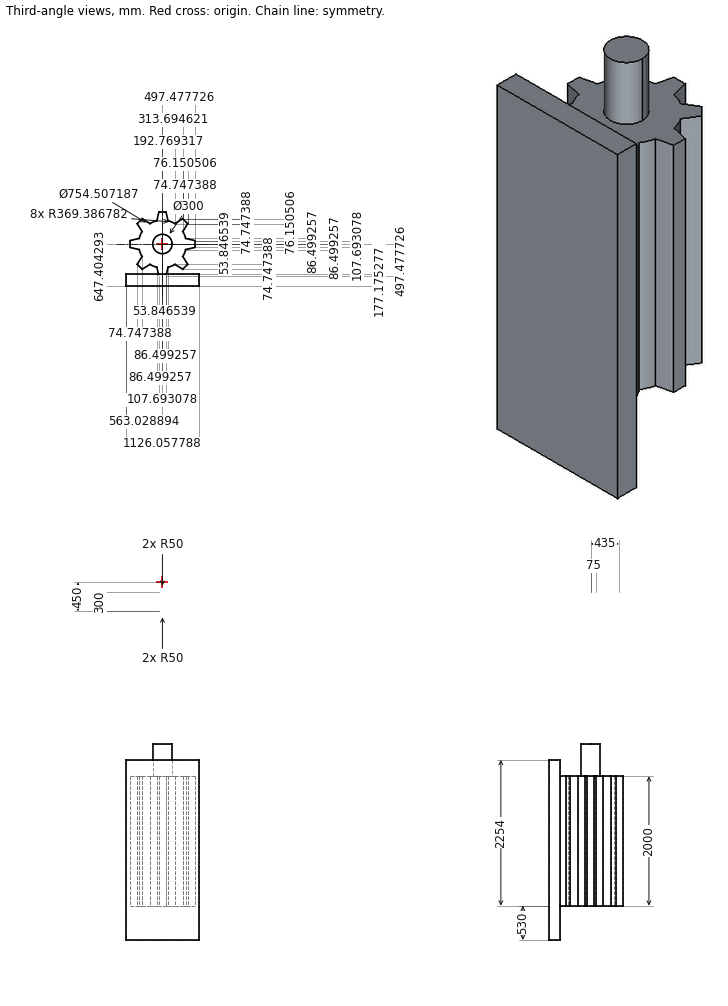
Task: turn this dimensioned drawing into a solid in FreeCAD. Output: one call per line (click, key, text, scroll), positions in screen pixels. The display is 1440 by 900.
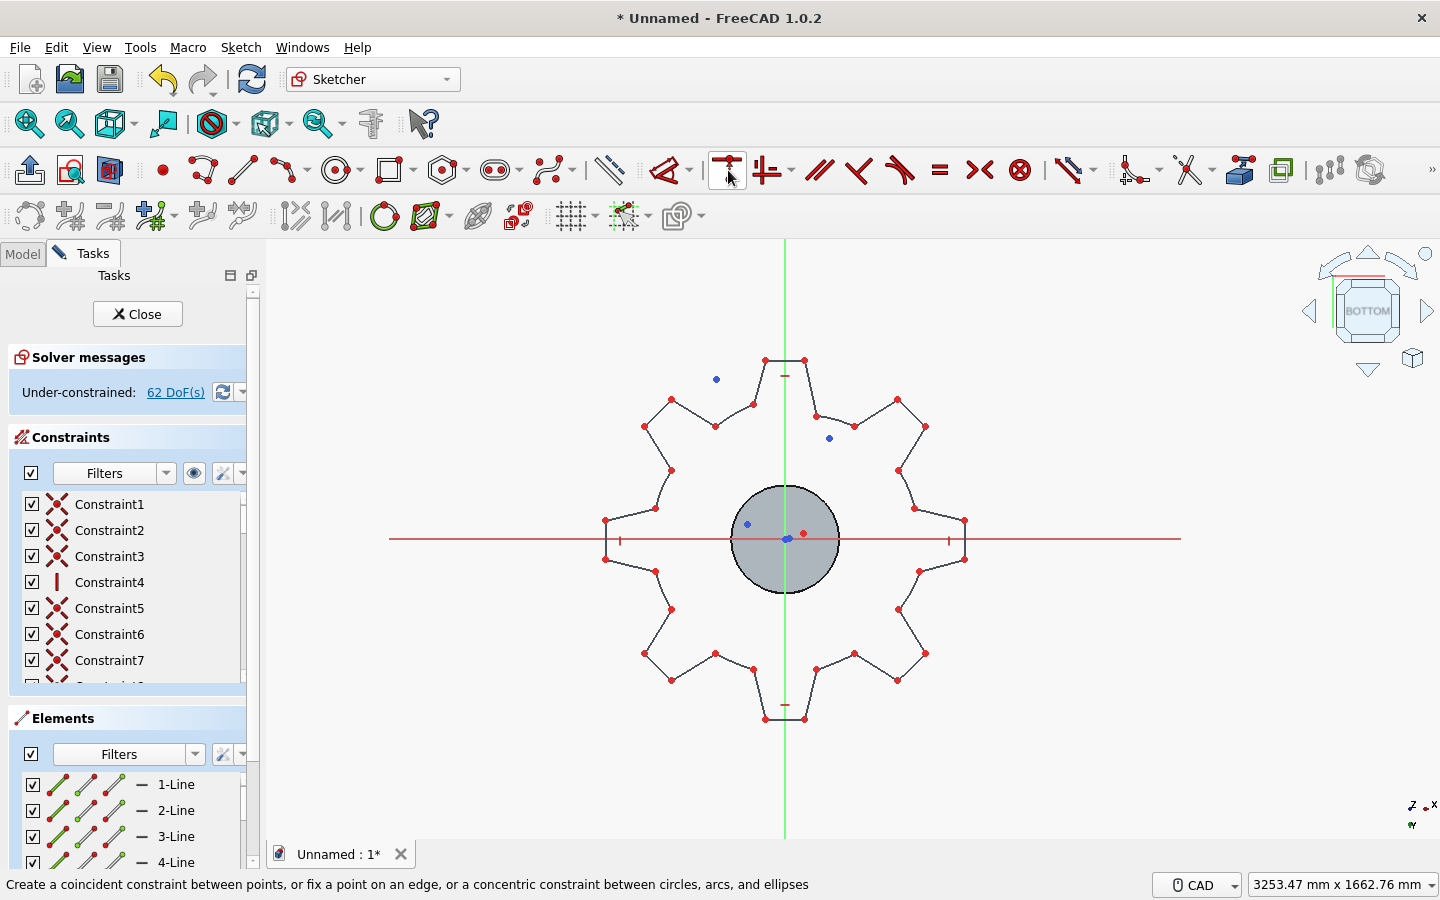
click(907, 599)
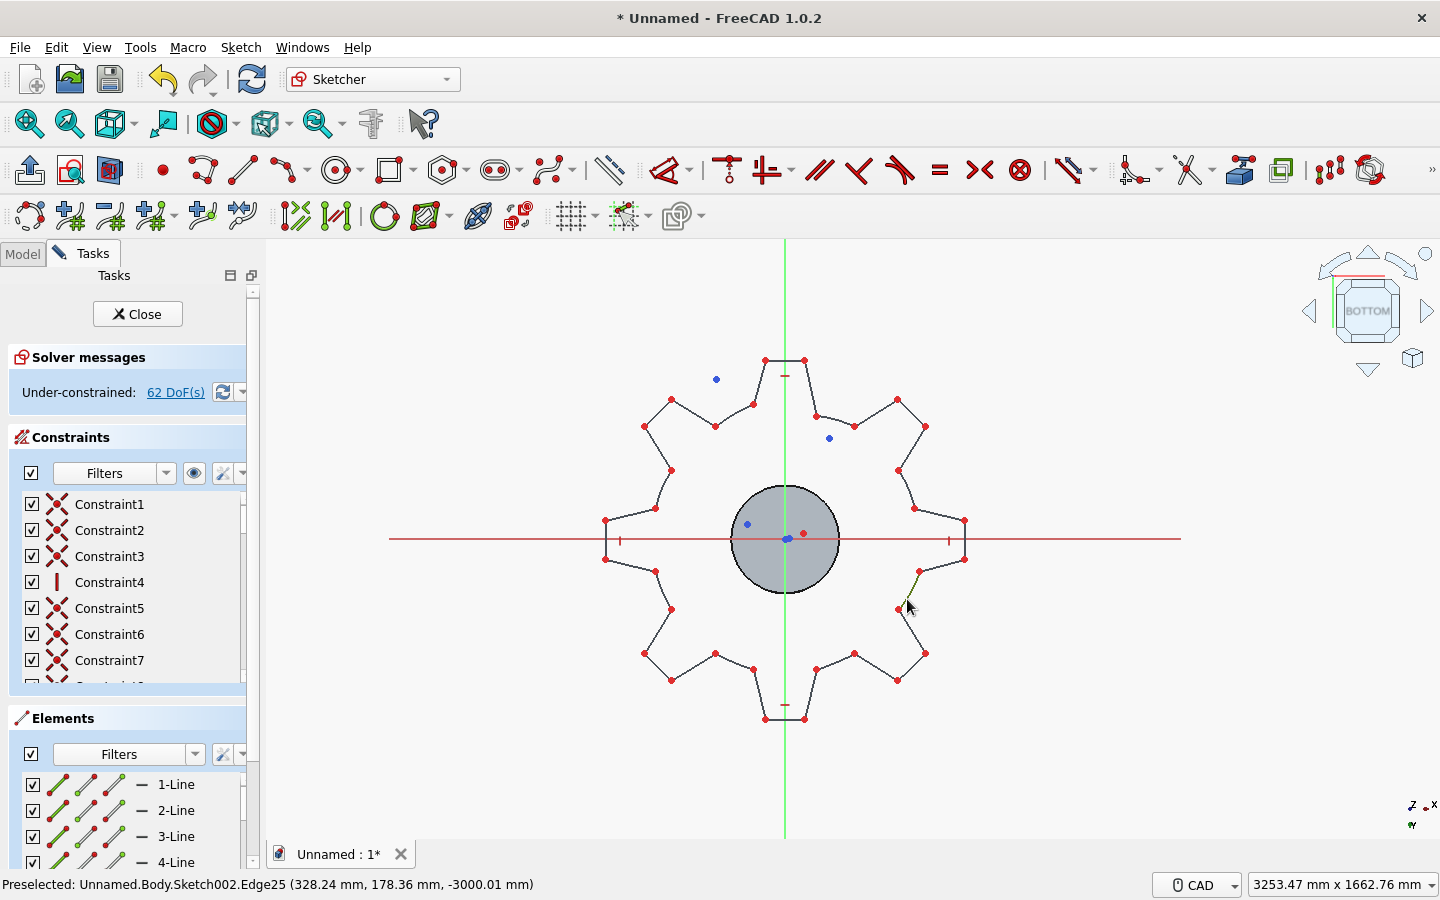
click(665, 481)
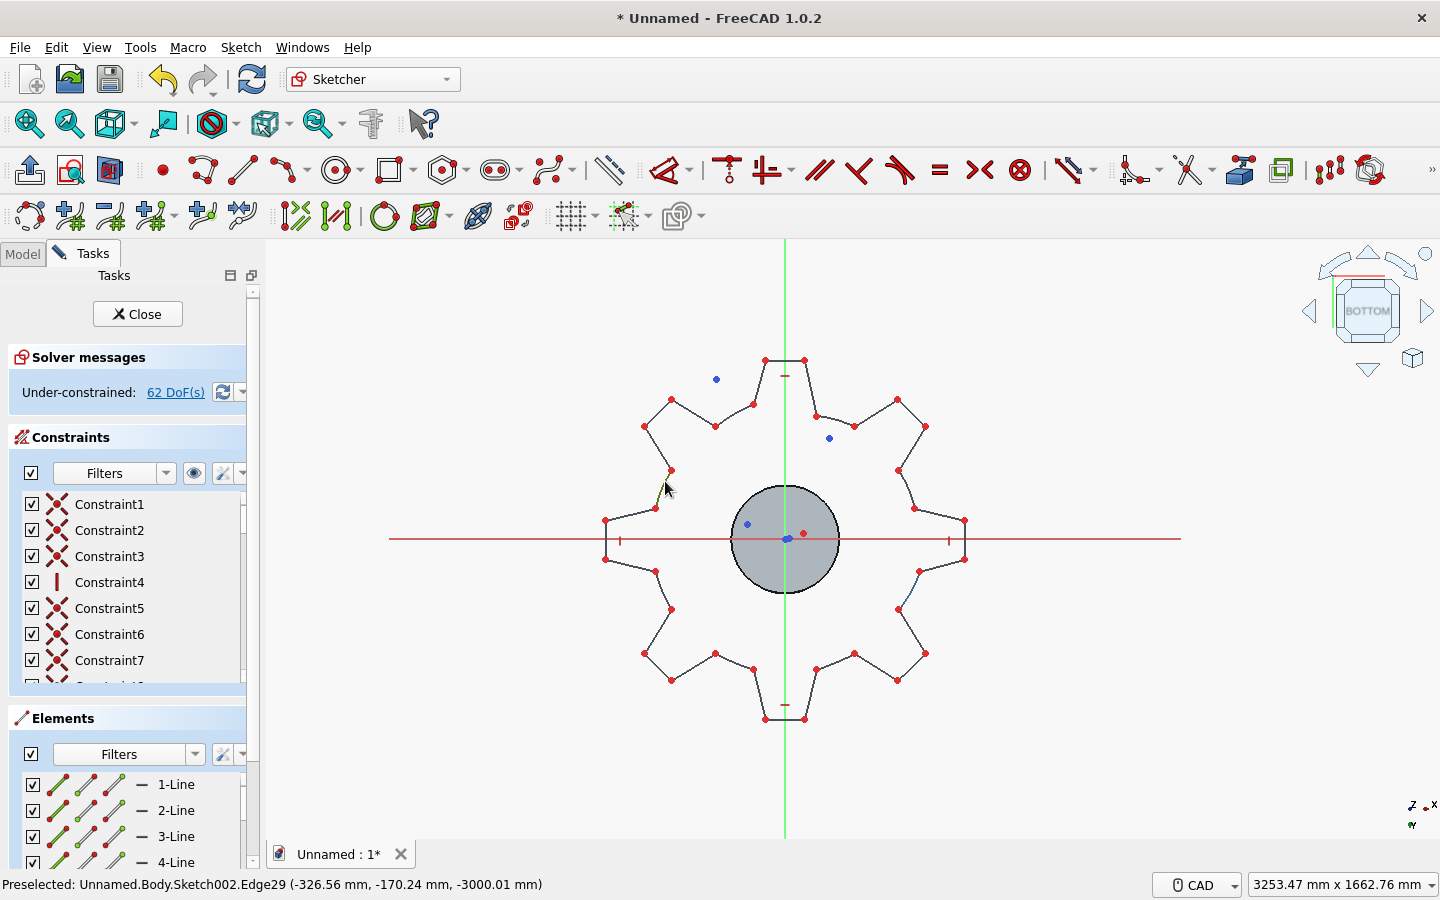
click(728, 170)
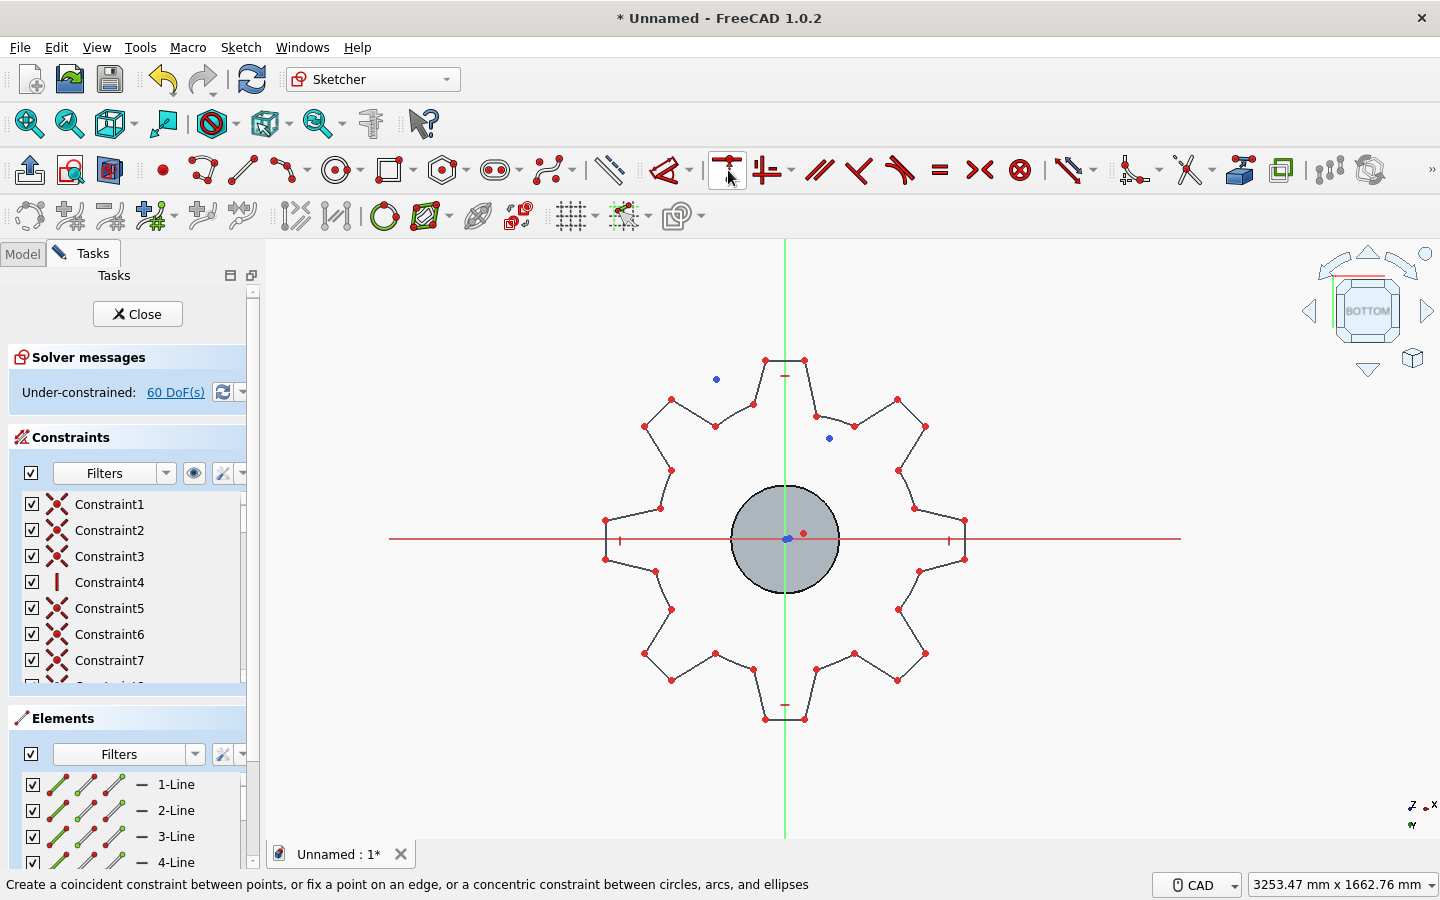
click(907, 599)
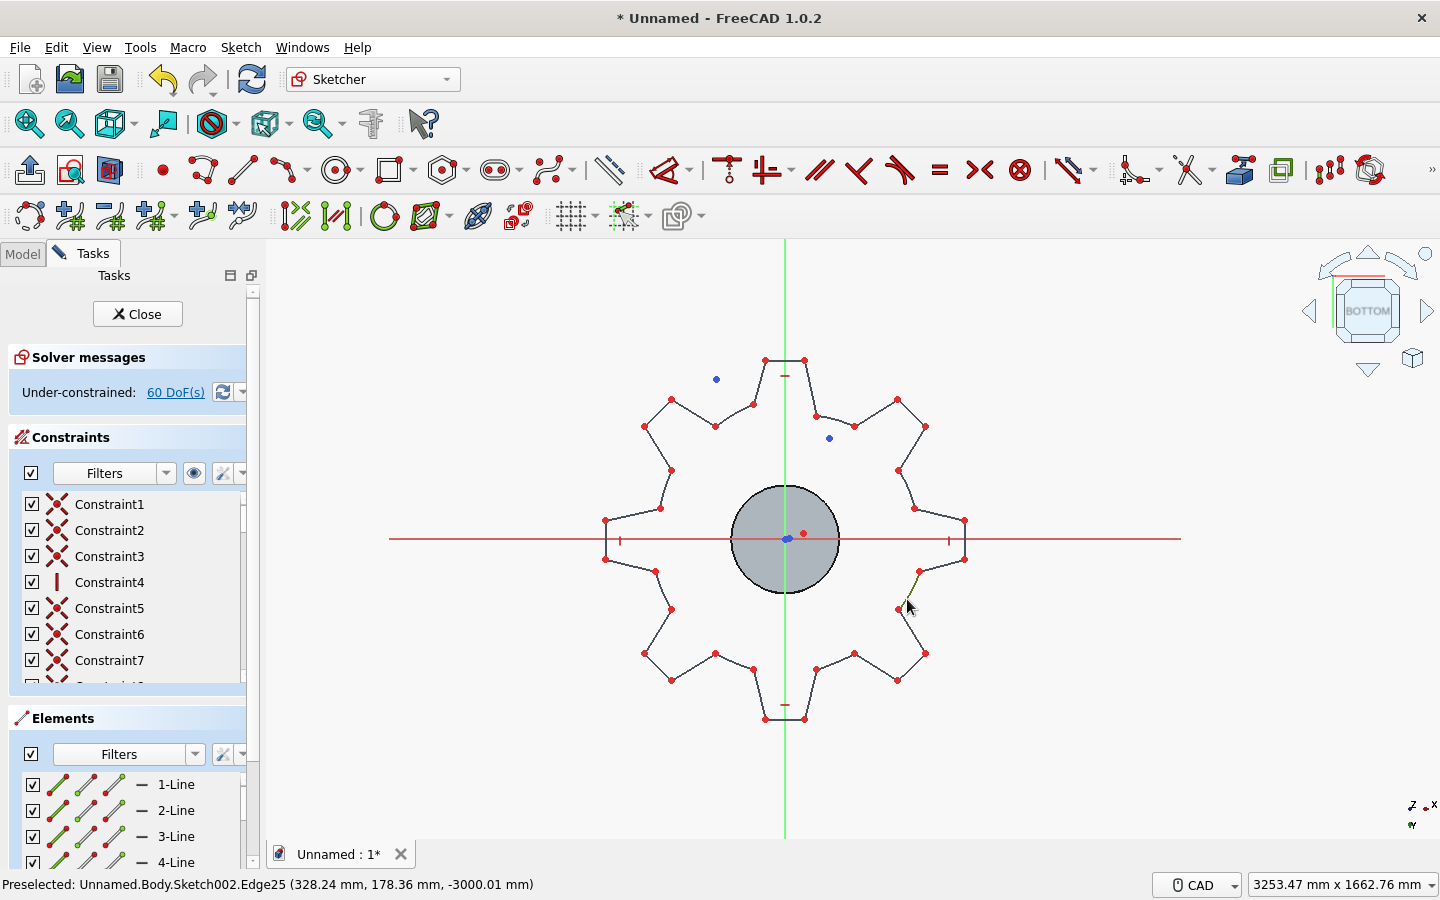
click(659, 584)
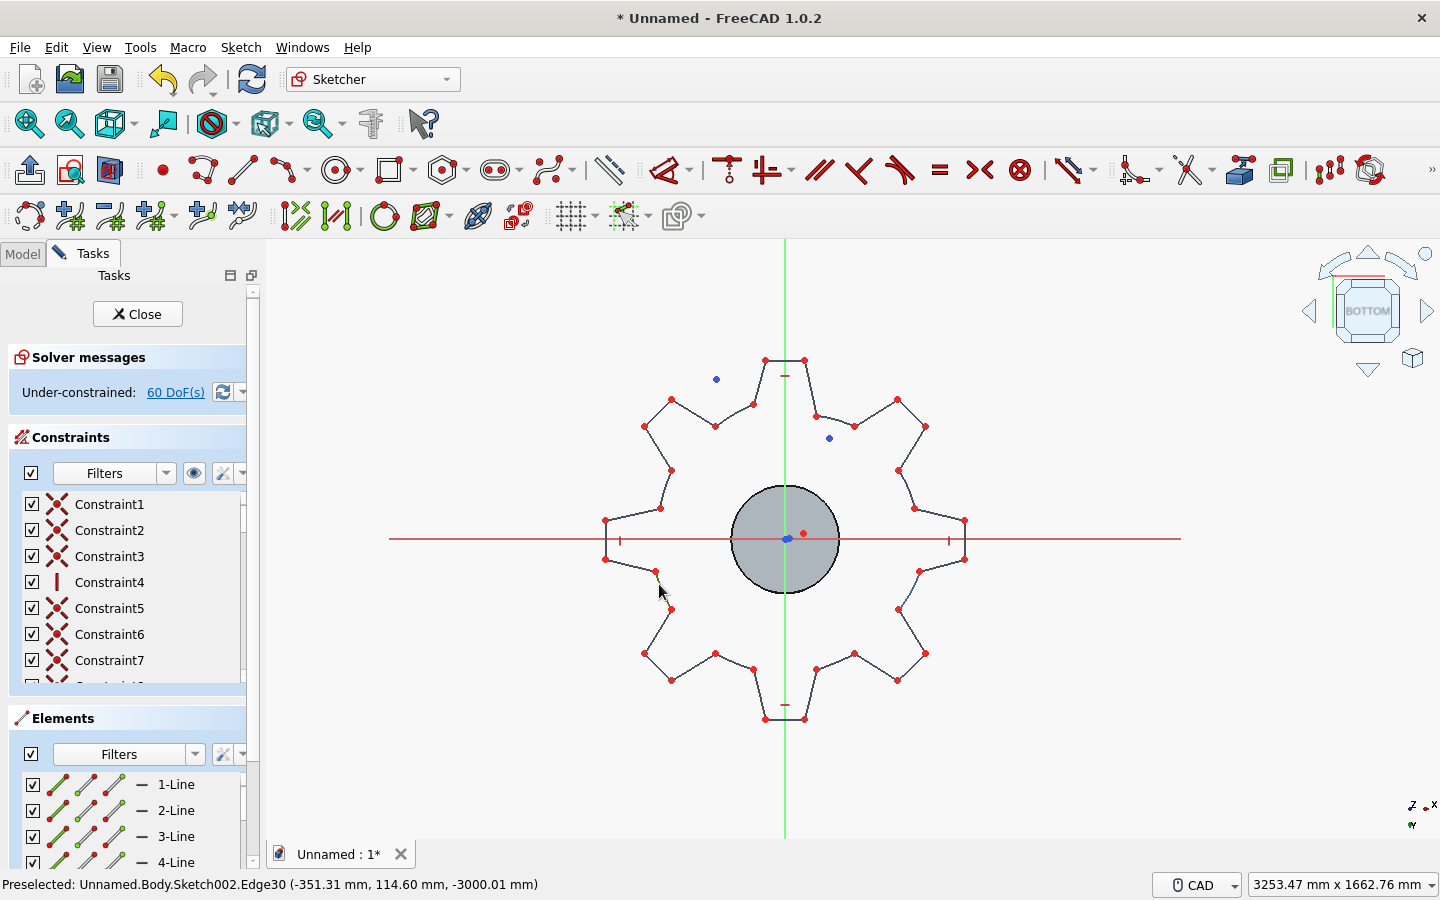
click(728, 170)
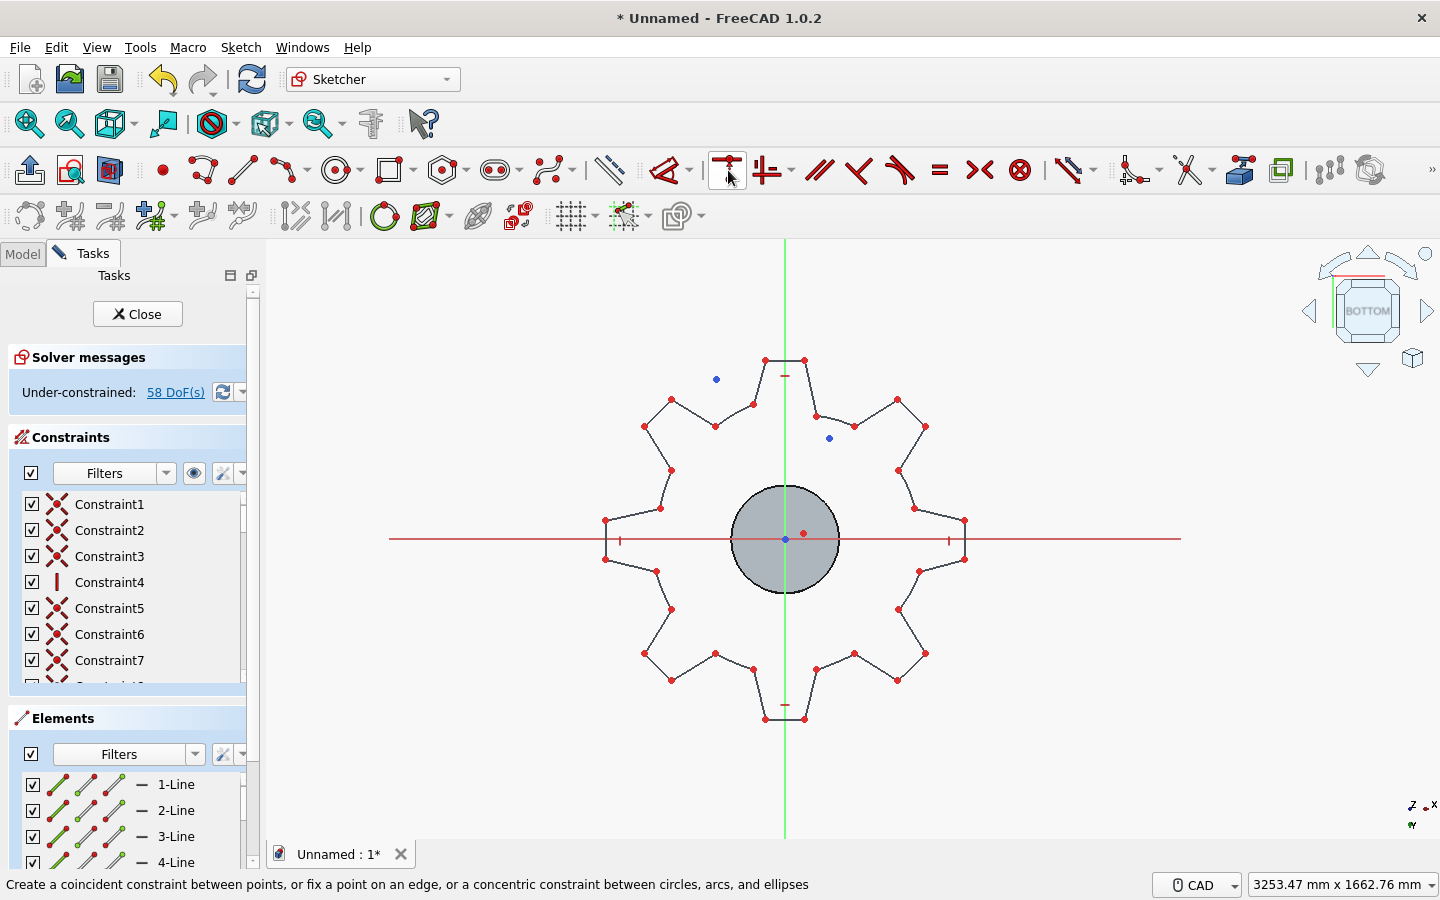
click(907, 599)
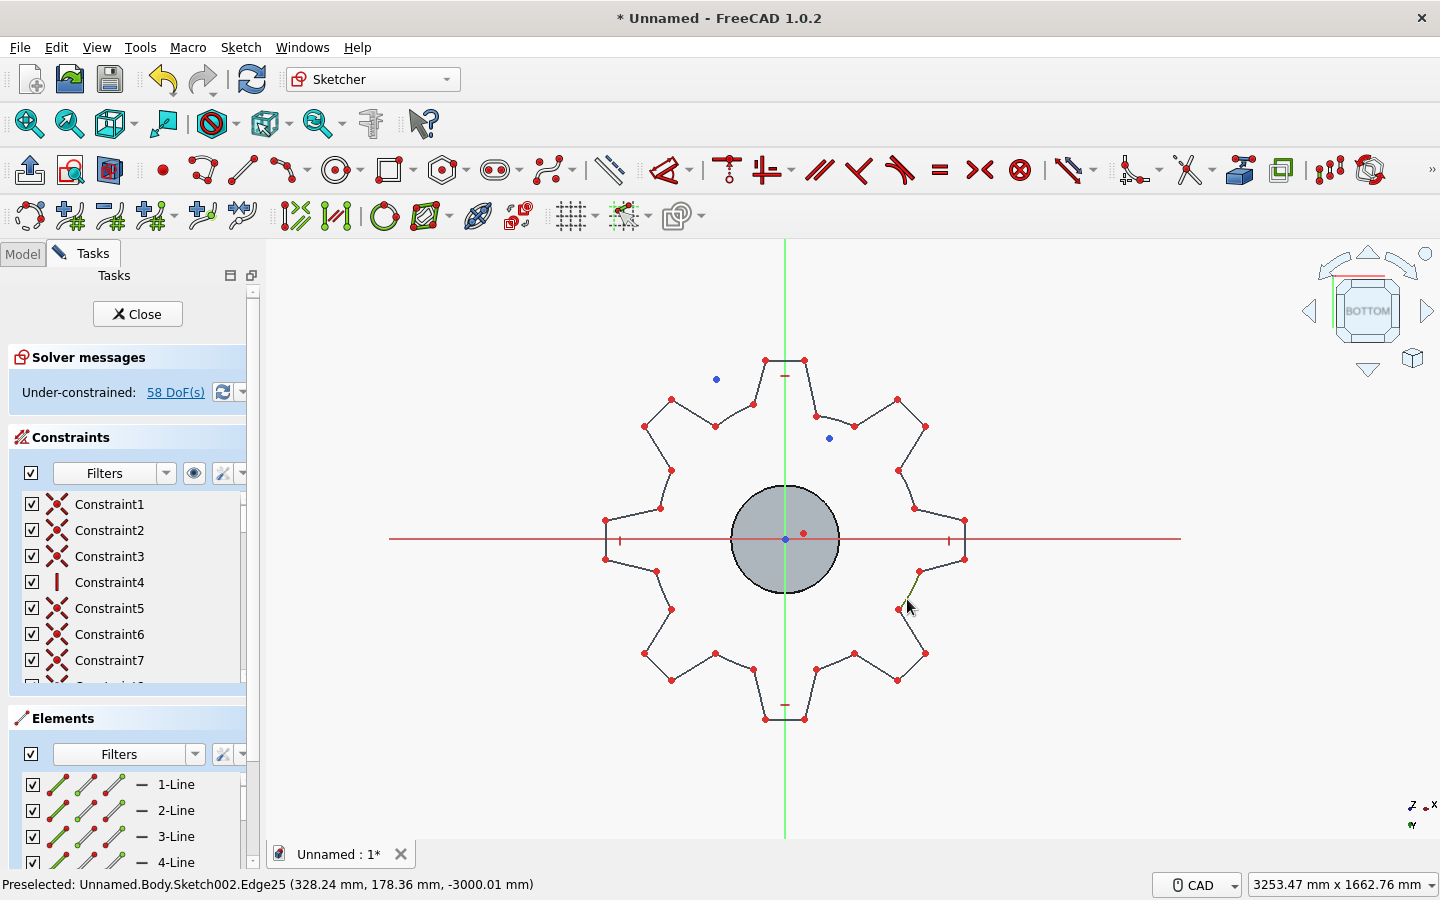
click(727, 659)